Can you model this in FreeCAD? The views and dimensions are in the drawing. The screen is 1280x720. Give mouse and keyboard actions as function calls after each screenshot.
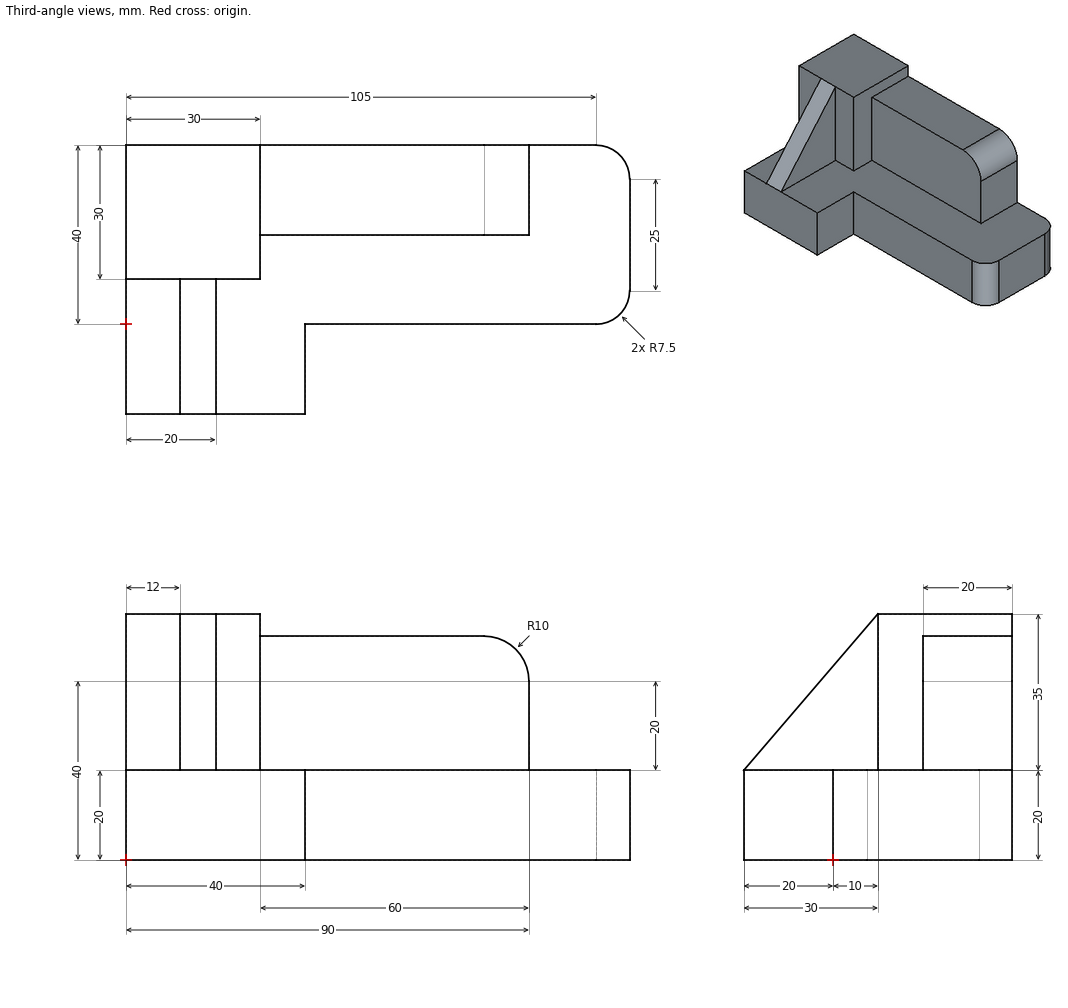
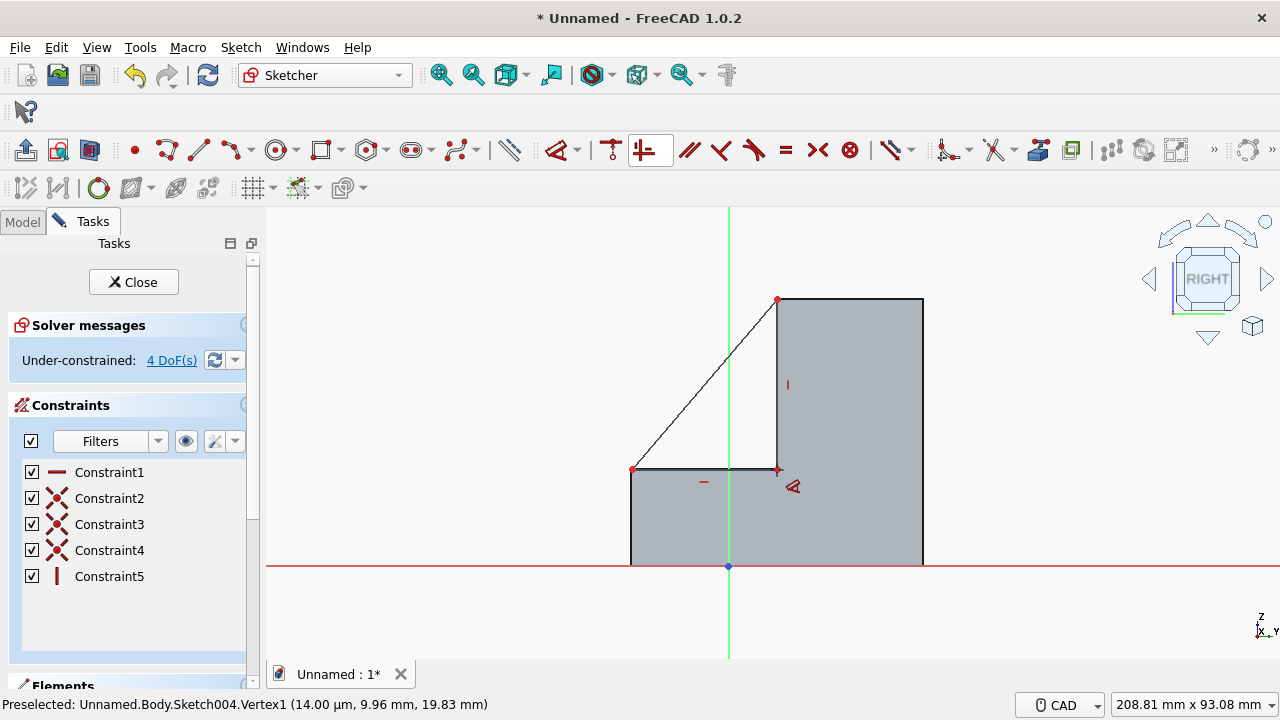
click(675, 470)
click(704, 504)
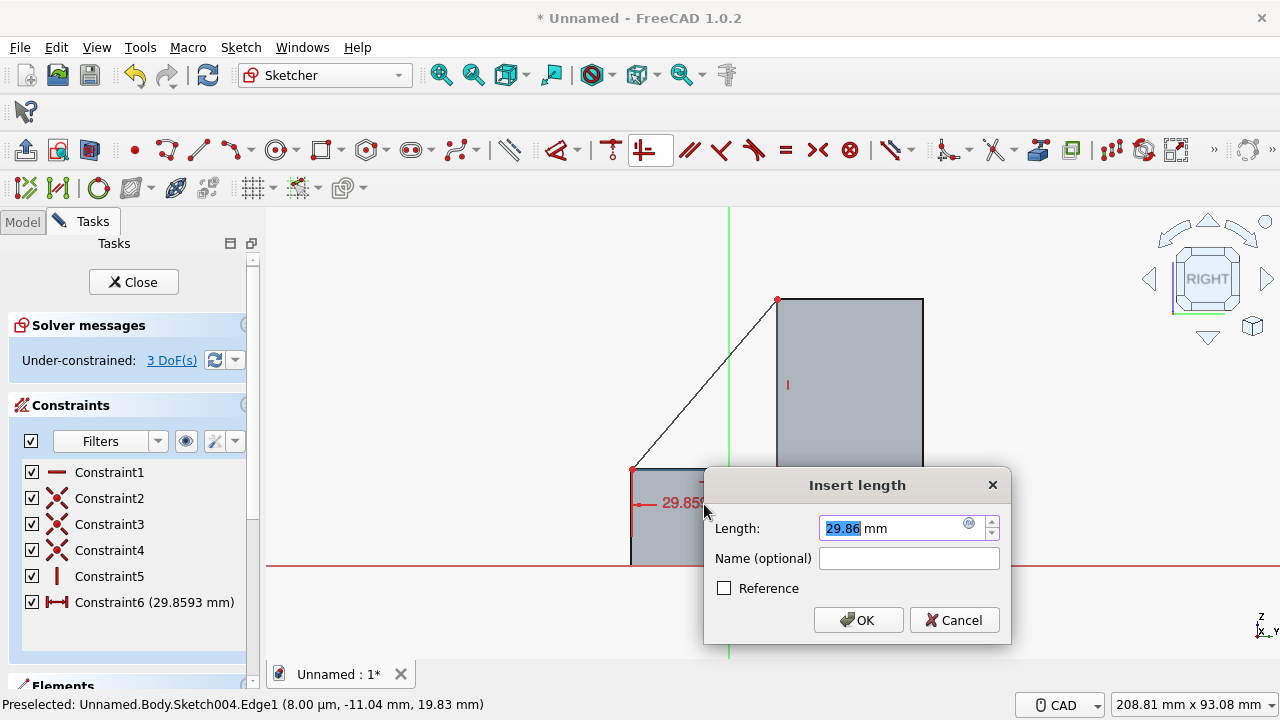
text(30)
key(Return)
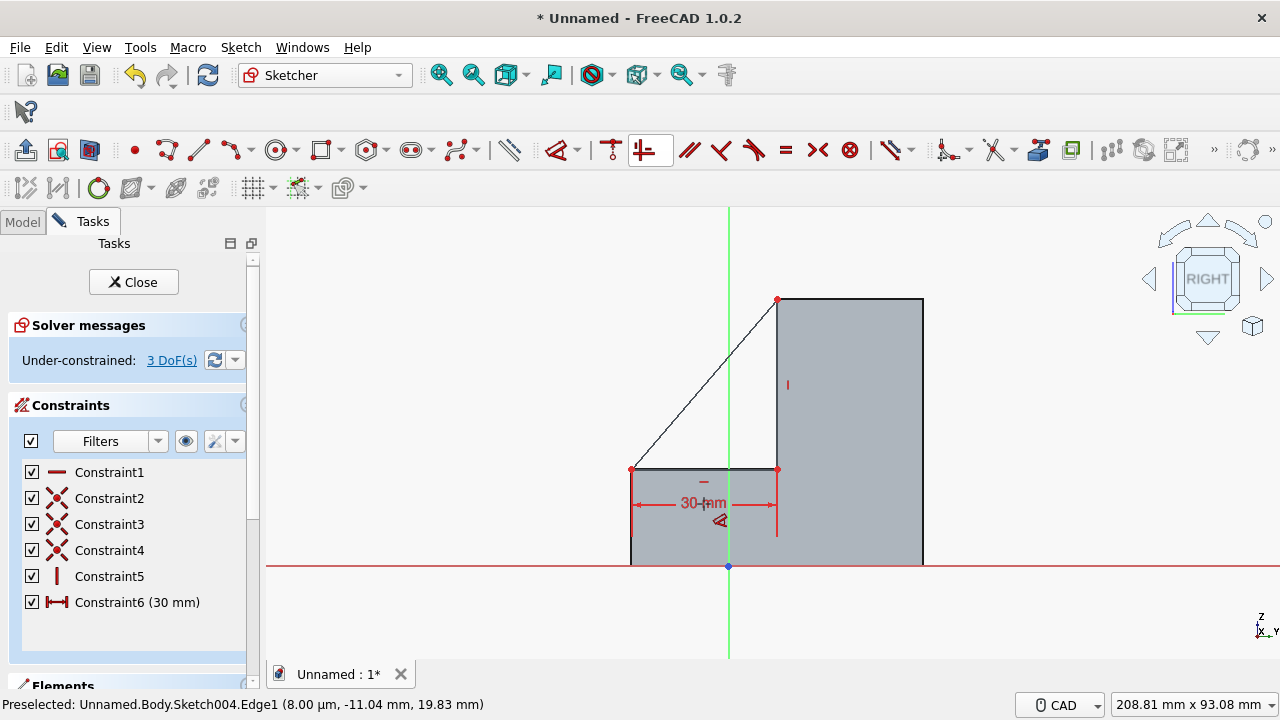
click(777, 351)
click(811, 385)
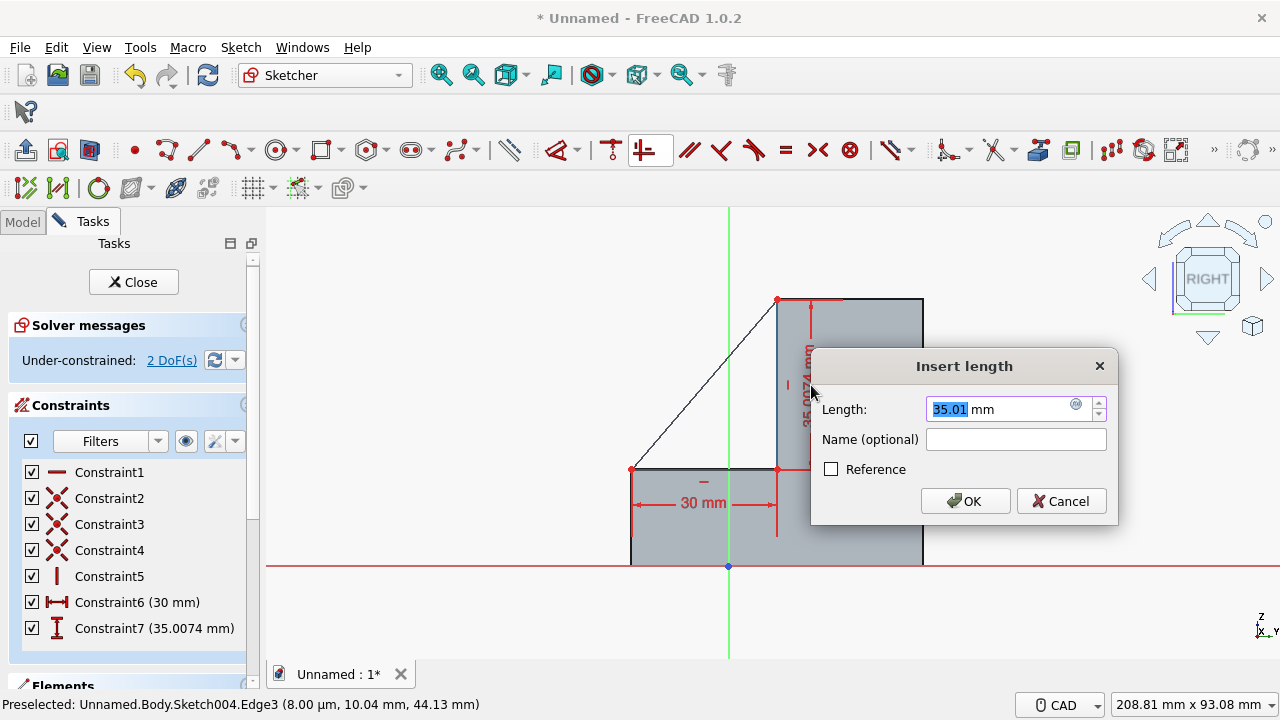
text(35)
key(Return)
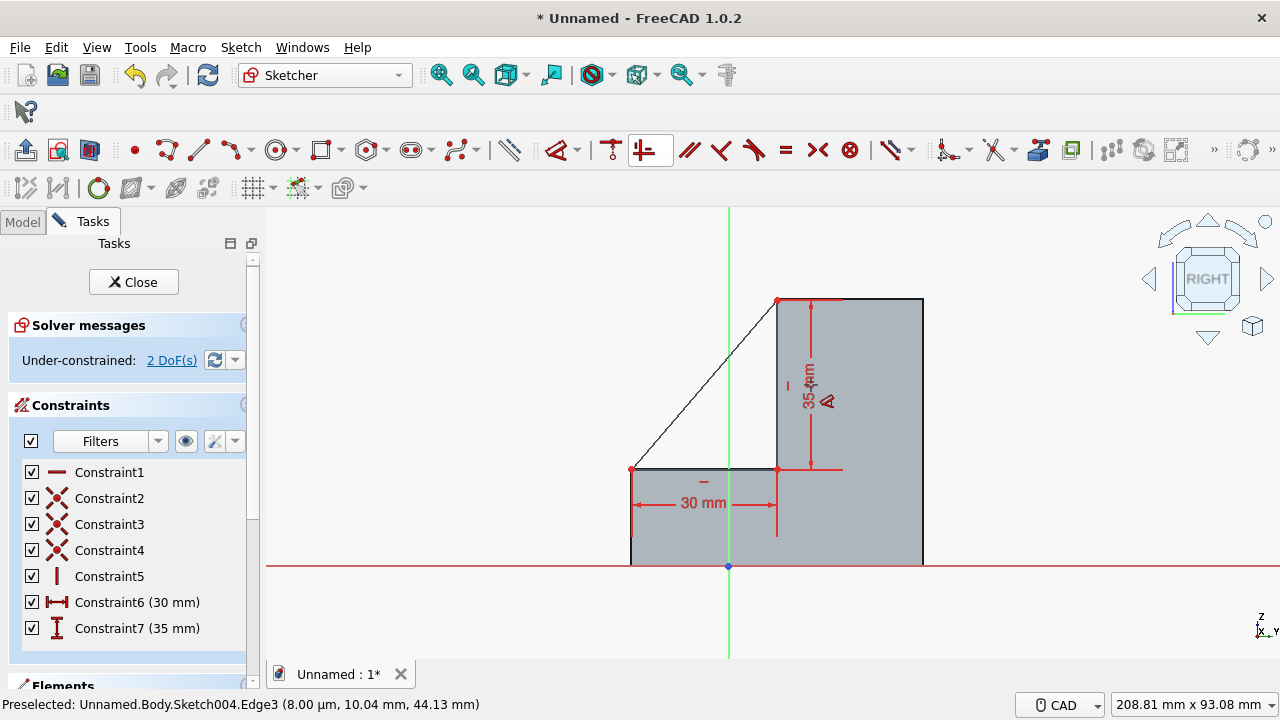
click(777, 470)
click(753, 600)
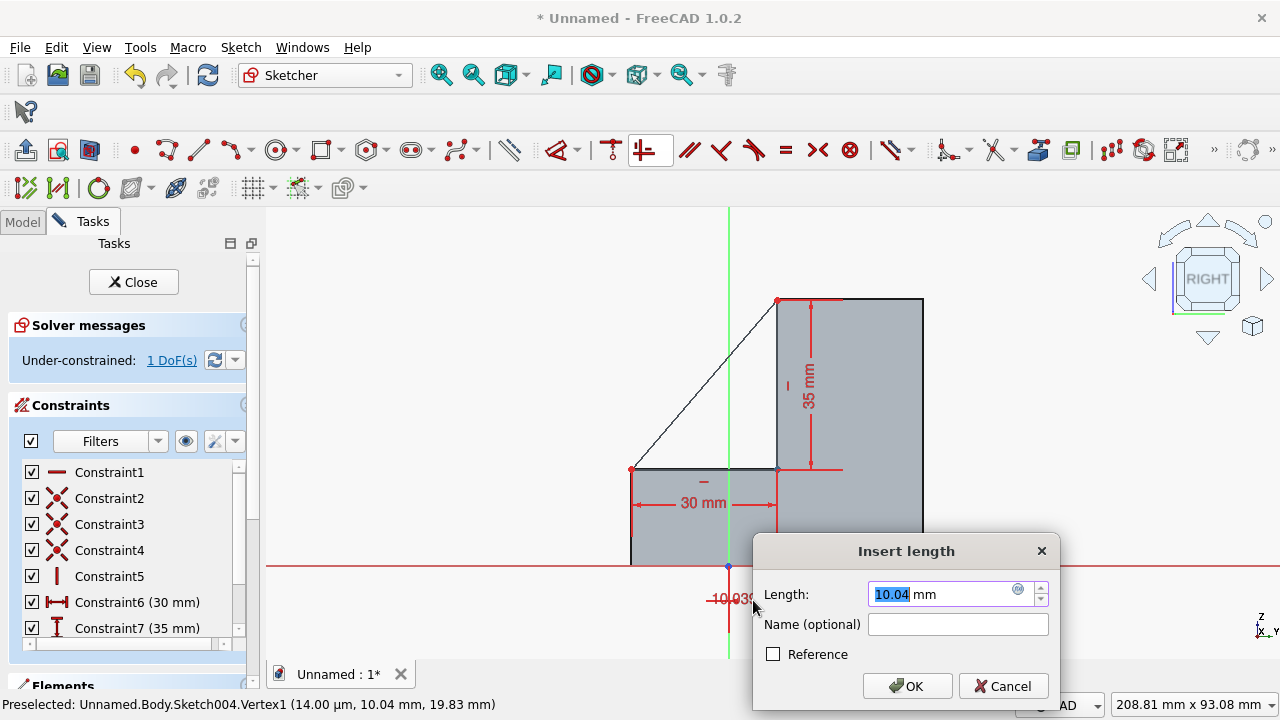
text(10)
key(Return)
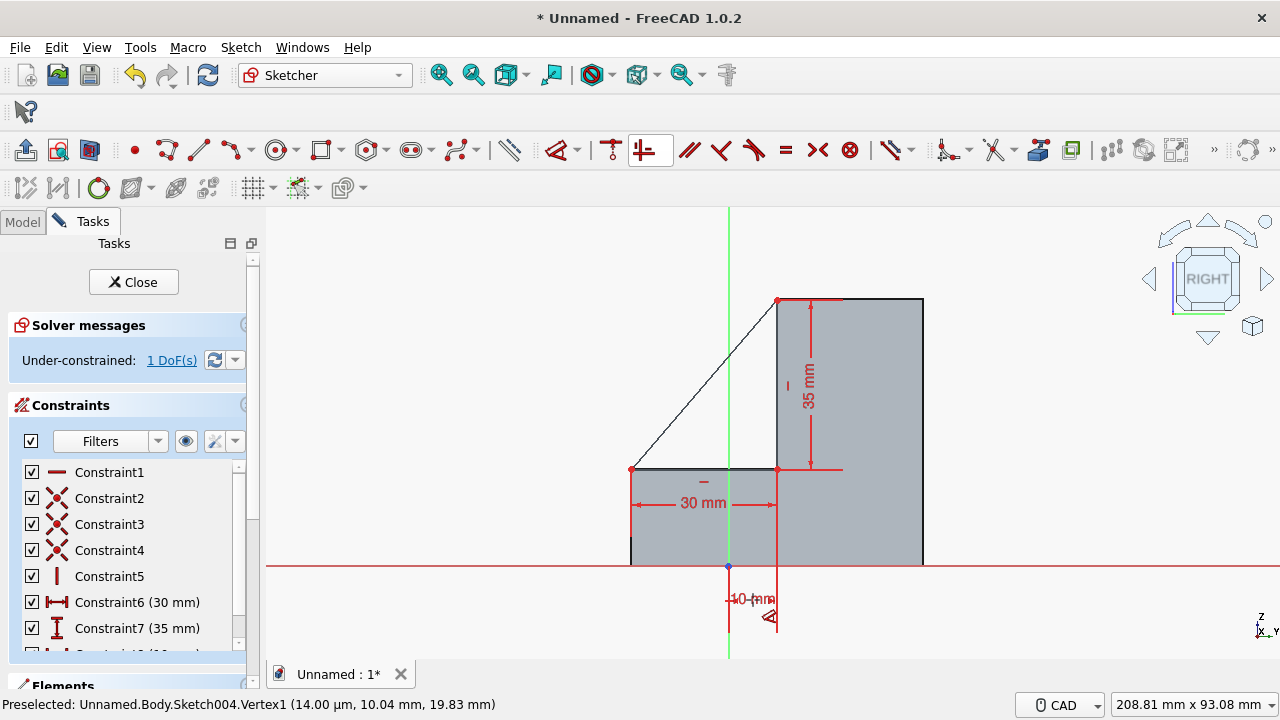
click(777, 470)
click(811, 518)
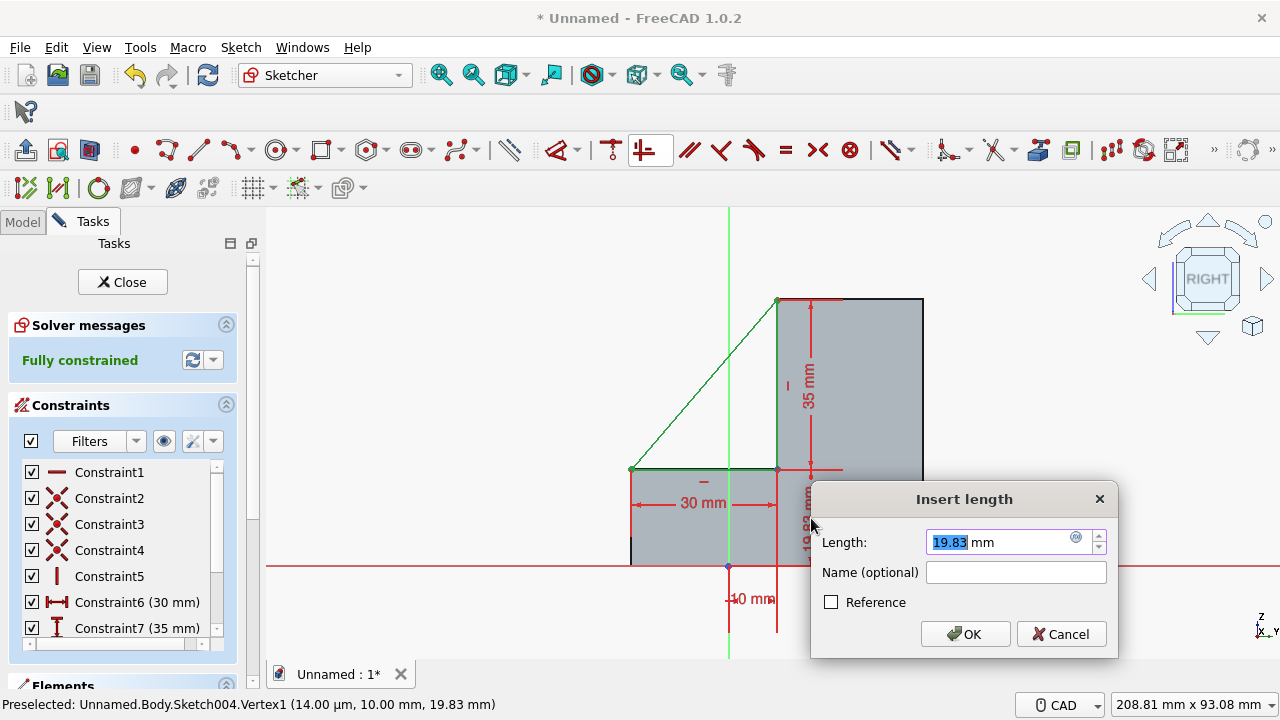
text(20)
key(Return)
key(Escape)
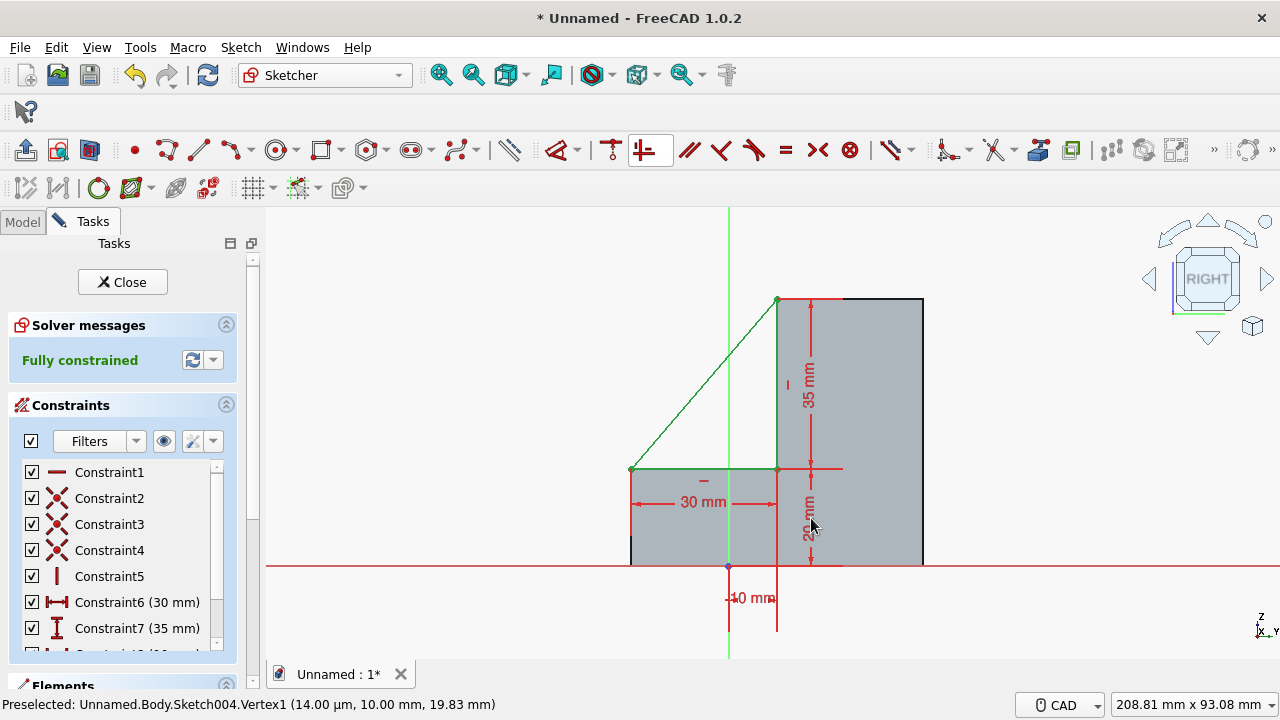
click(123, 282)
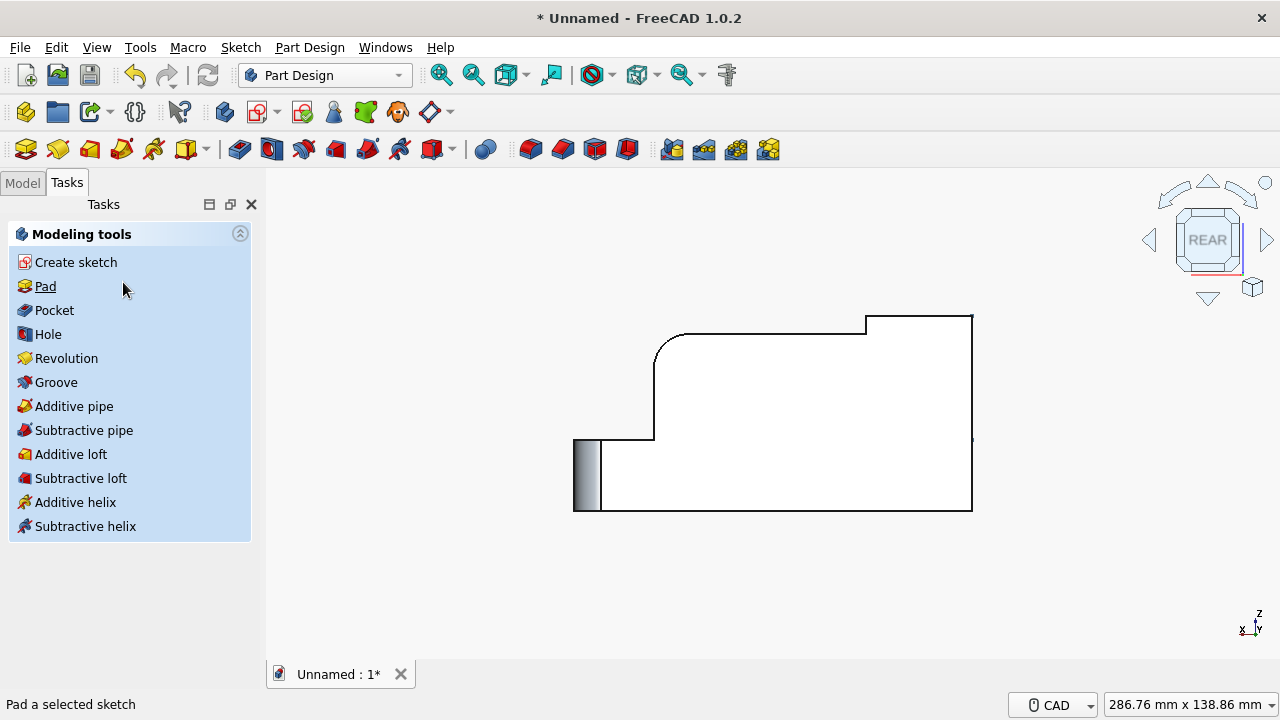
click(26, 150)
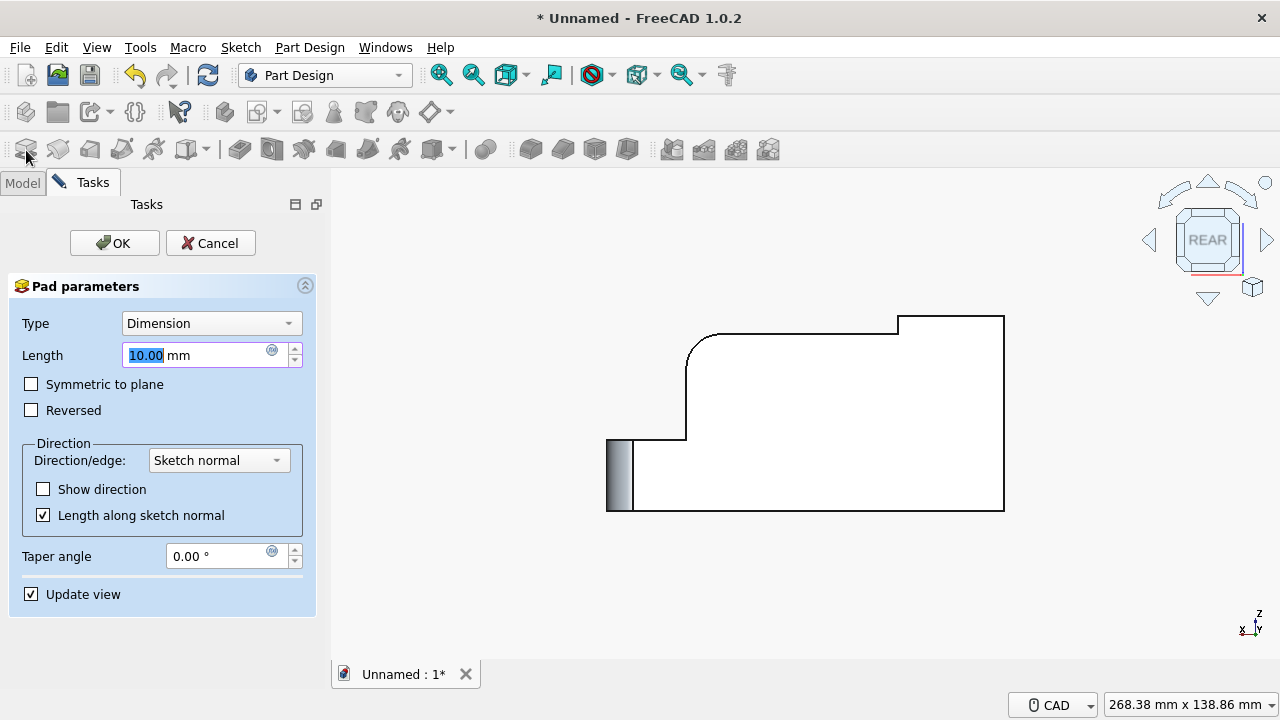
text(20)
key(Tab)